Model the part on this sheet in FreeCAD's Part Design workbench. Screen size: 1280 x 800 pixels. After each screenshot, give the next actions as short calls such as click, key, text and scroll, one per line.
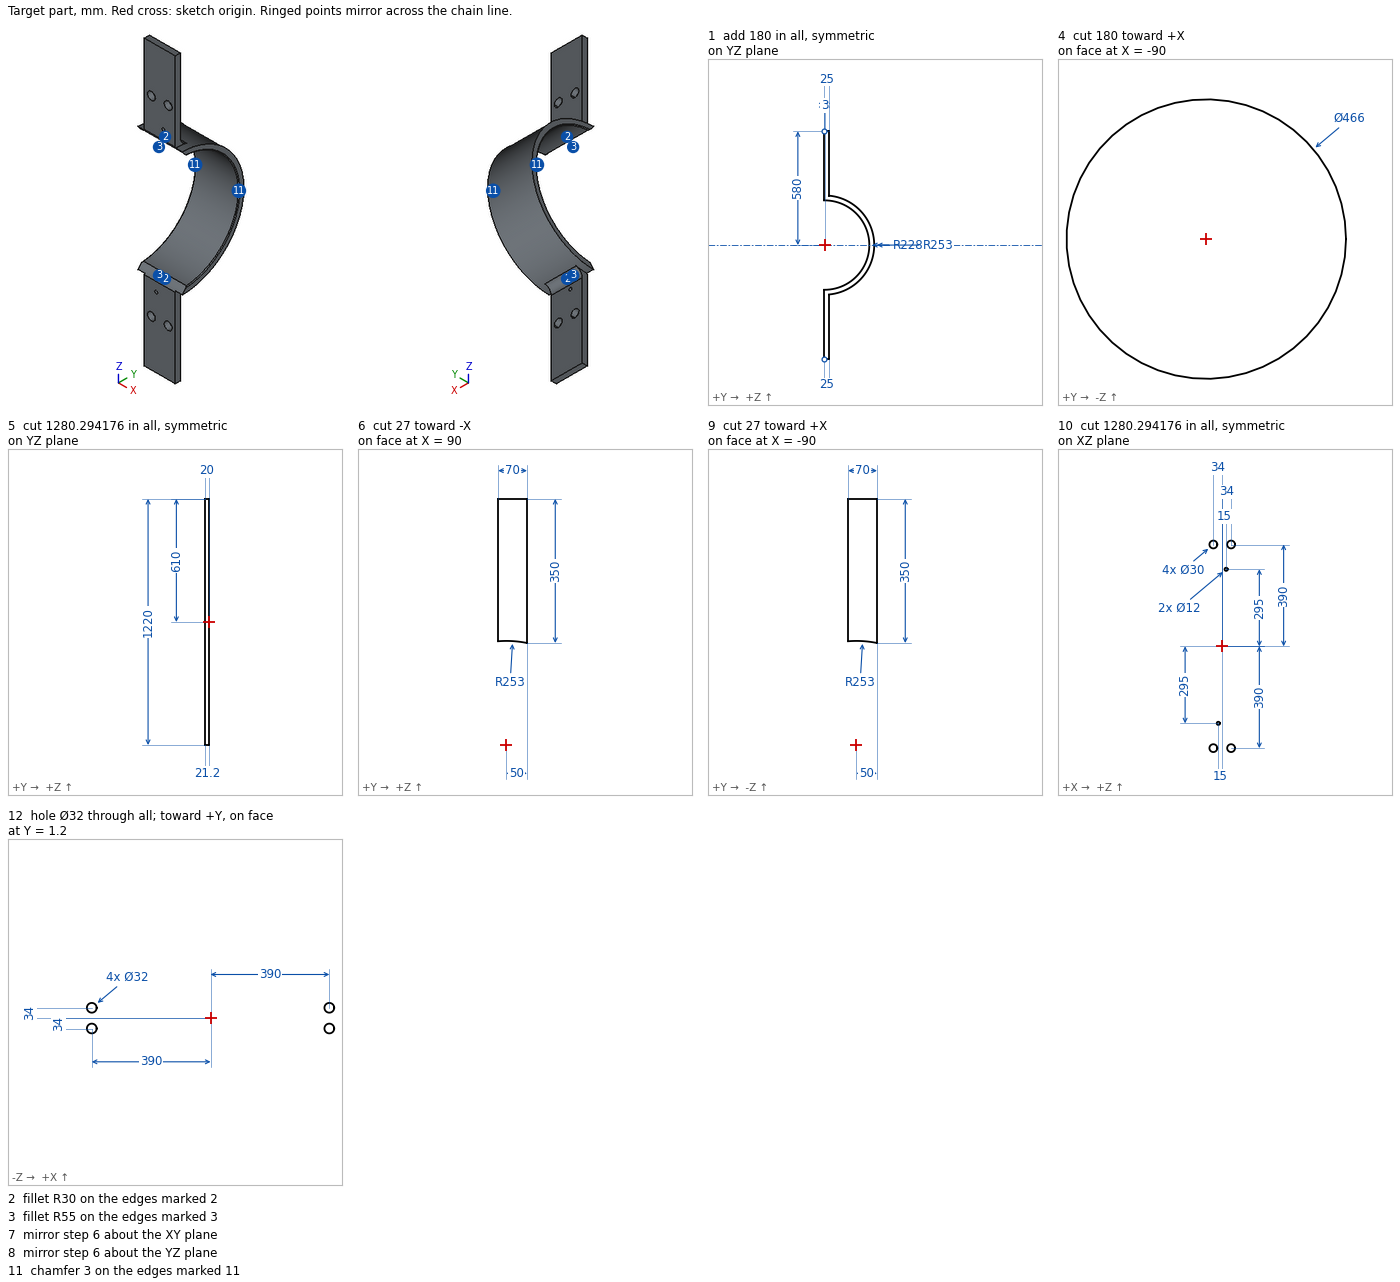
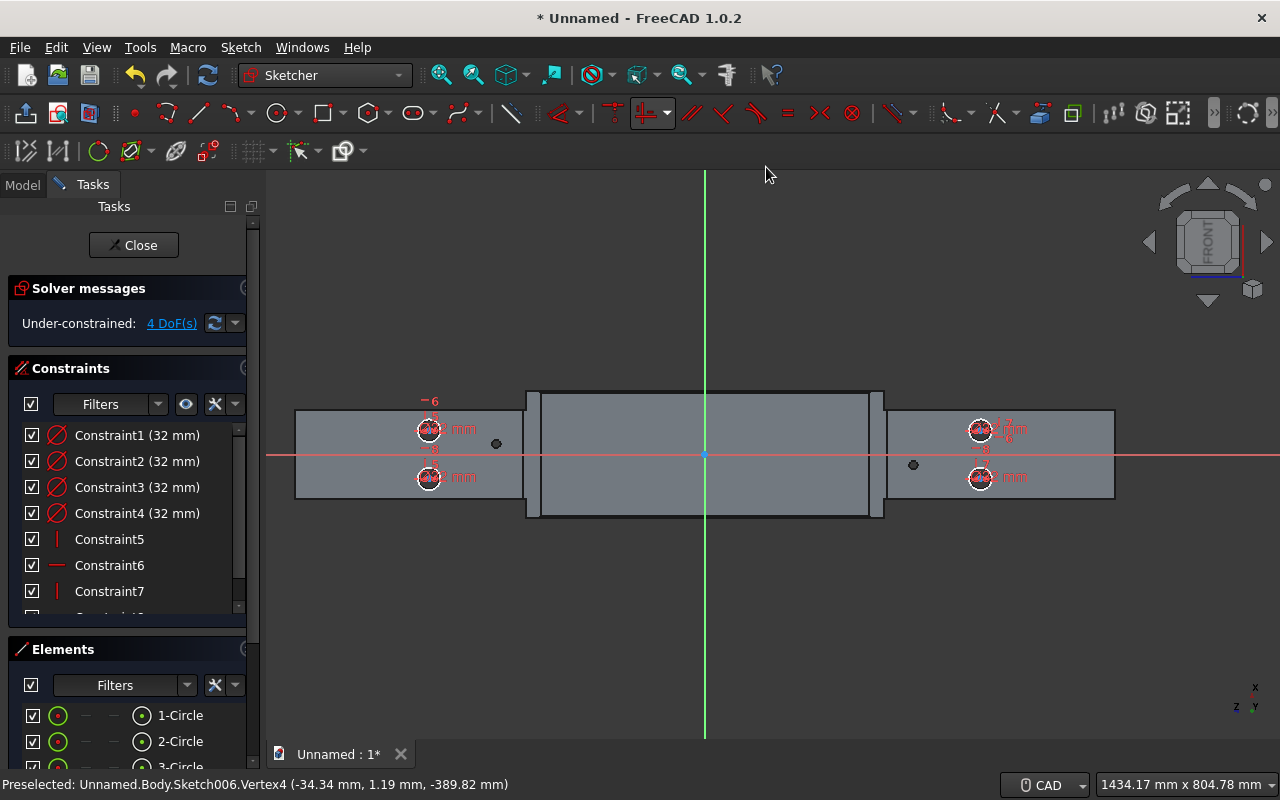
click(558, 114)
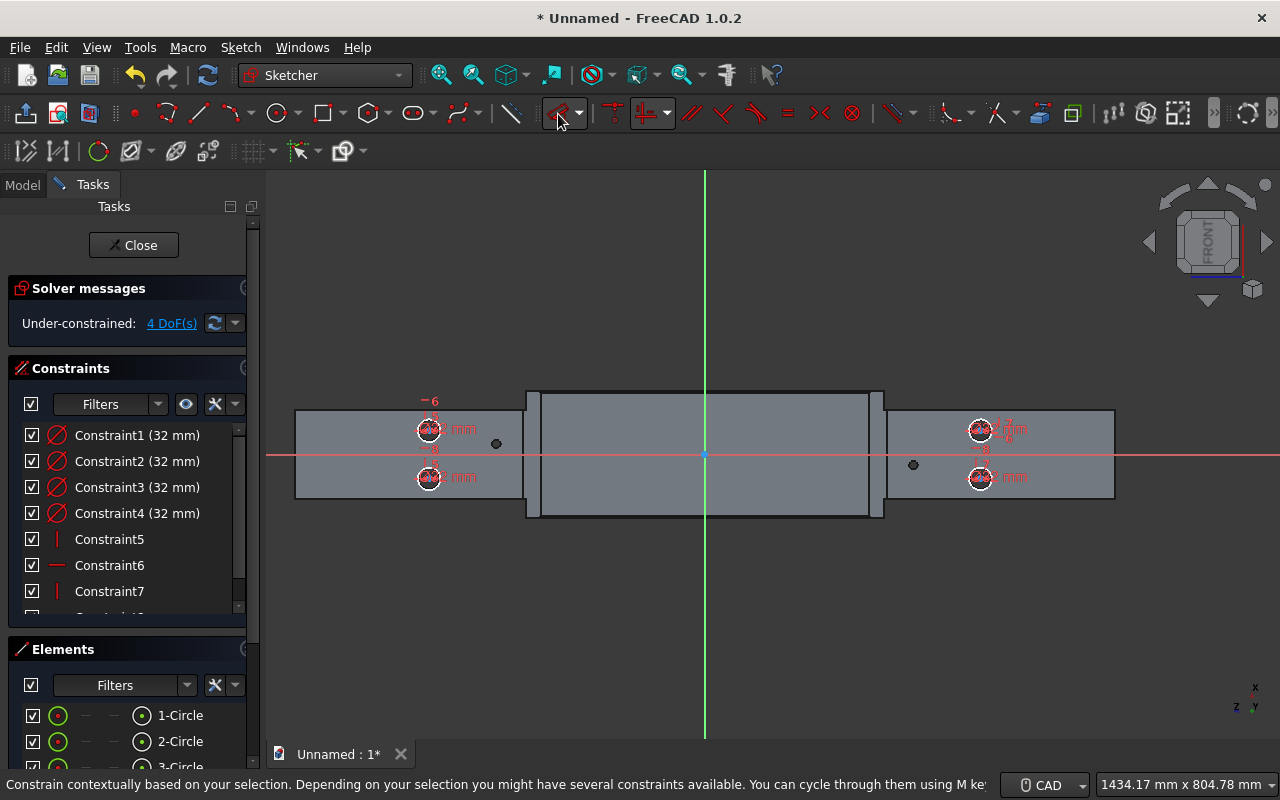
scroll(429, 479, up, 3)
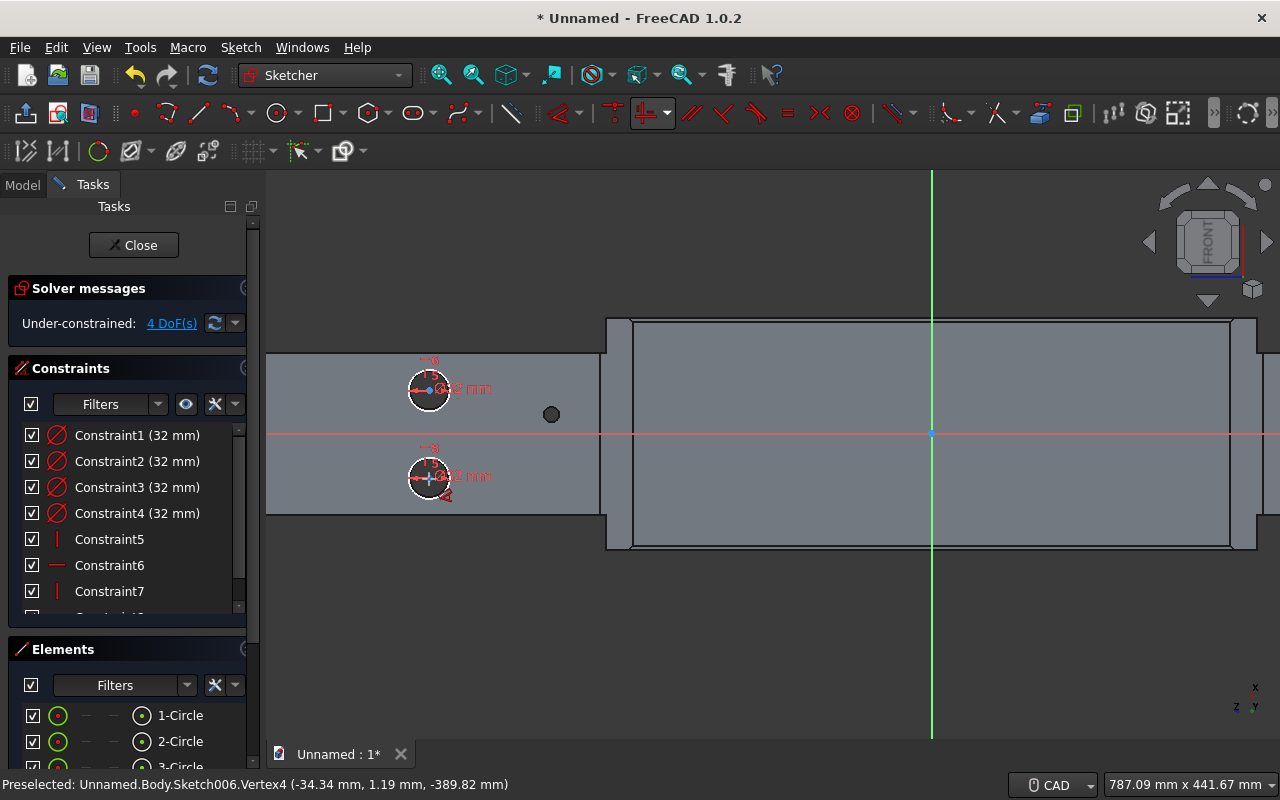
click(429, 478)
click(395, 456)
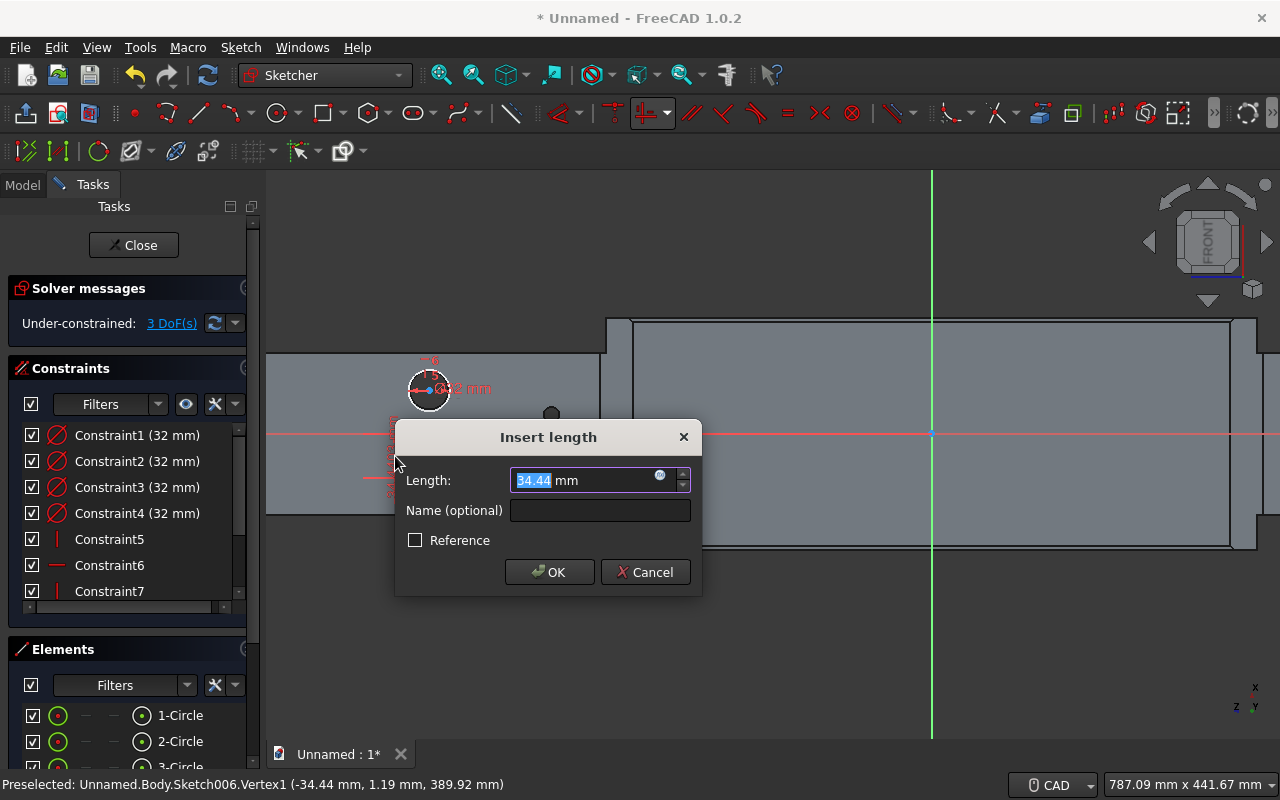
text(34)
key(Return)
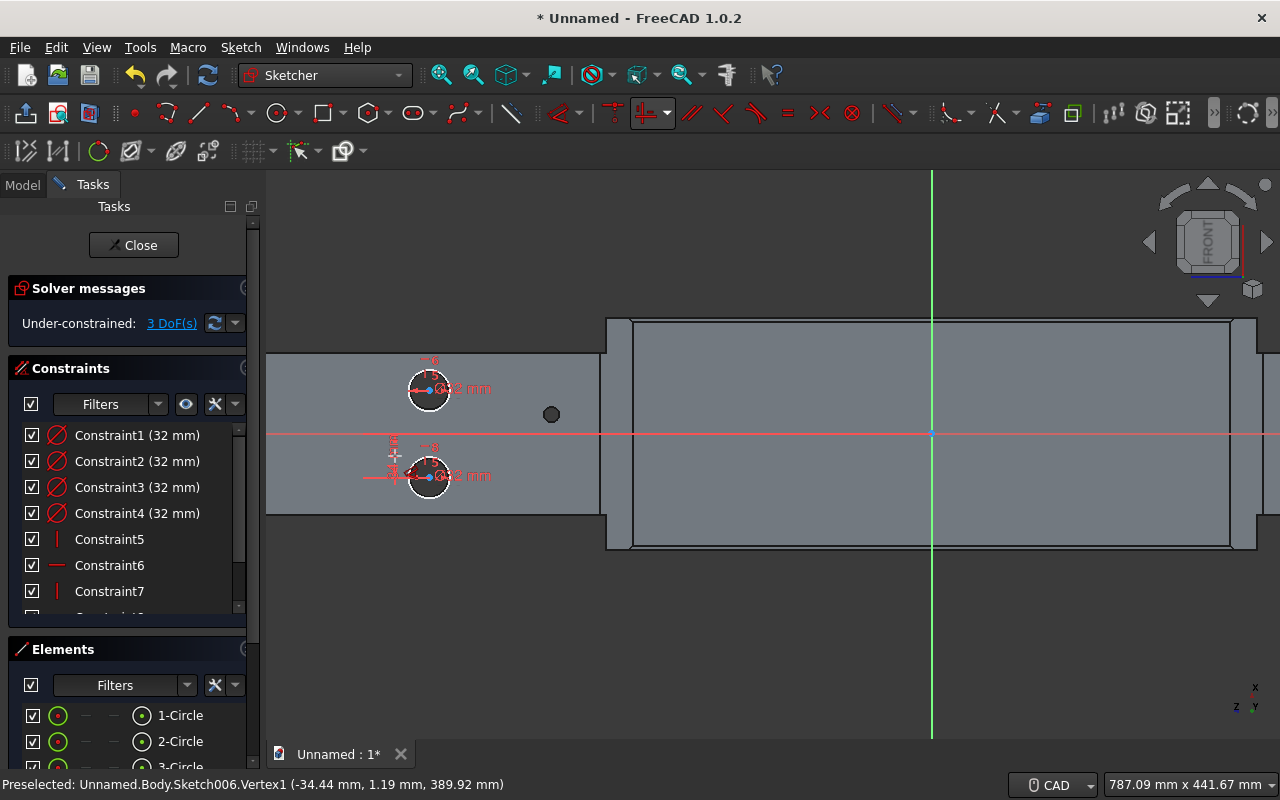
click(429, 391)
click(395, 412)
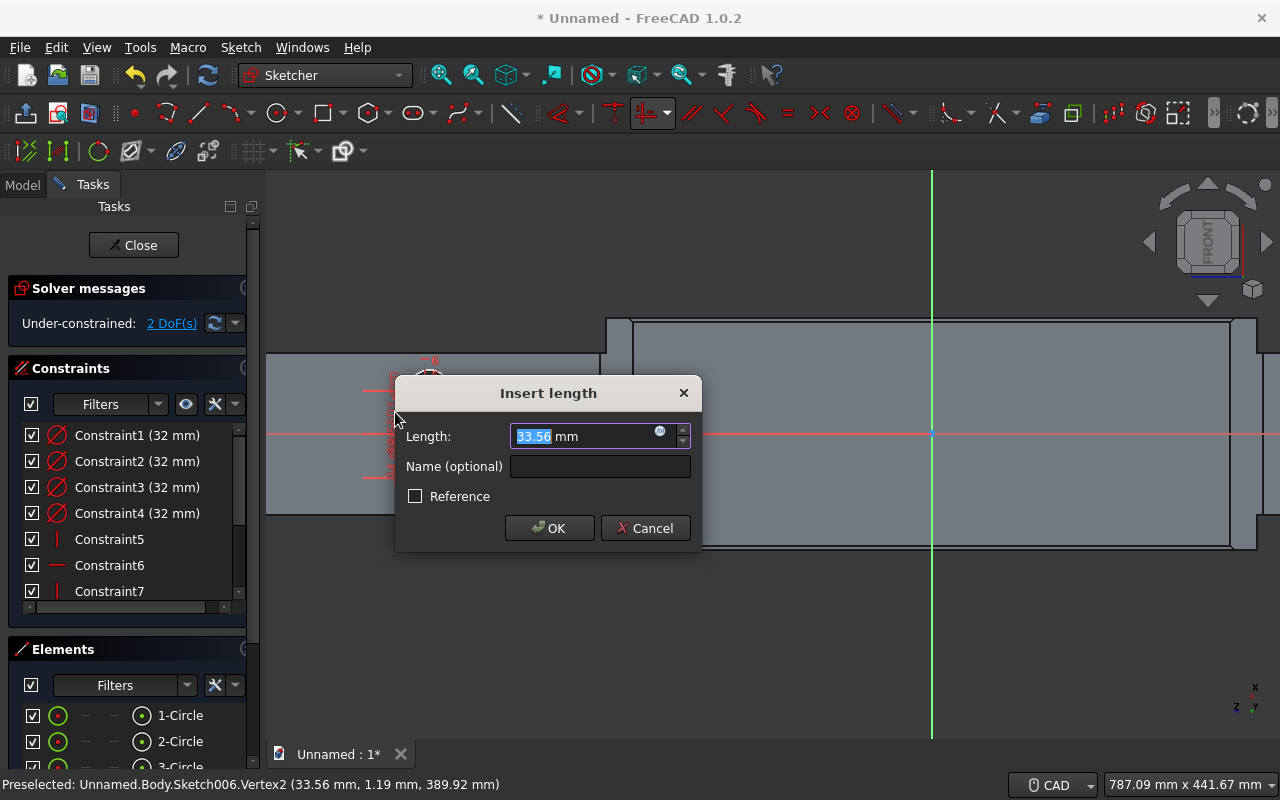
text(34)
key(Return)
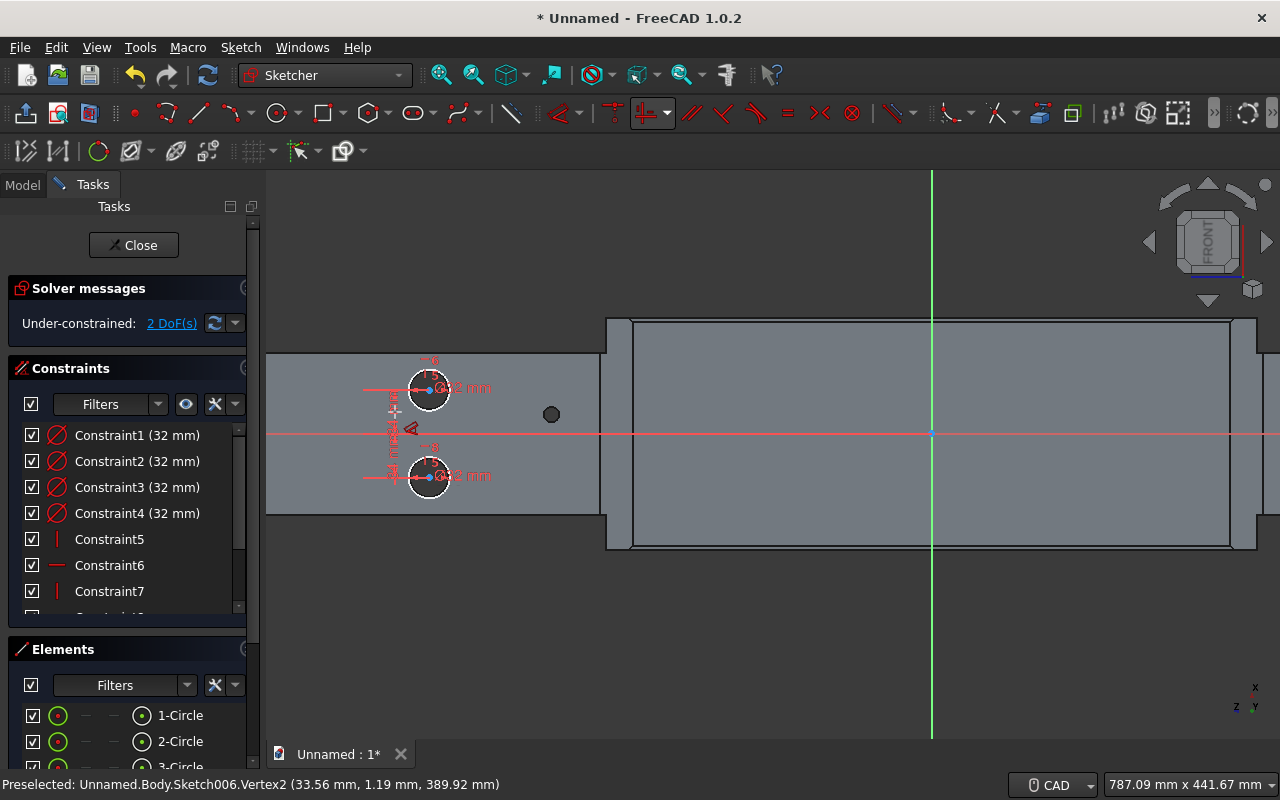
click(429, 478)
click(680, 512)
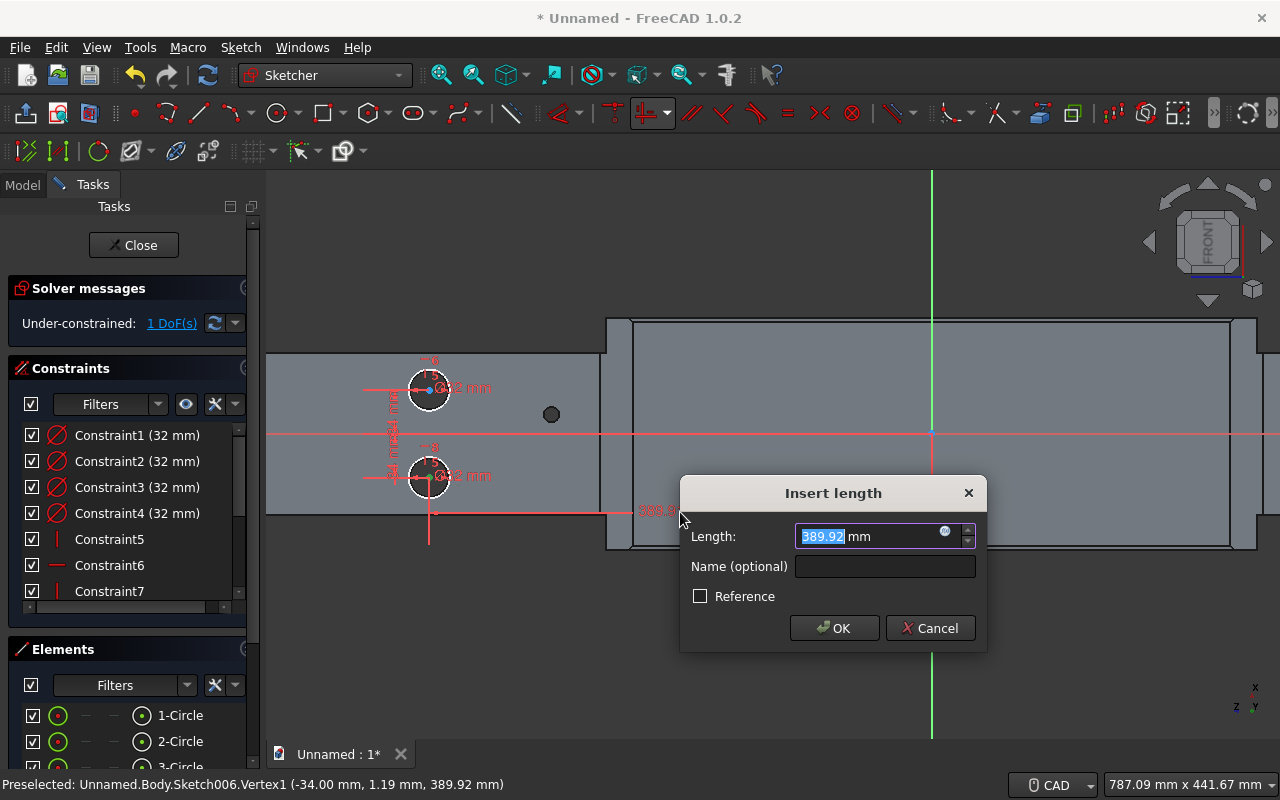
text(390)
key(Return)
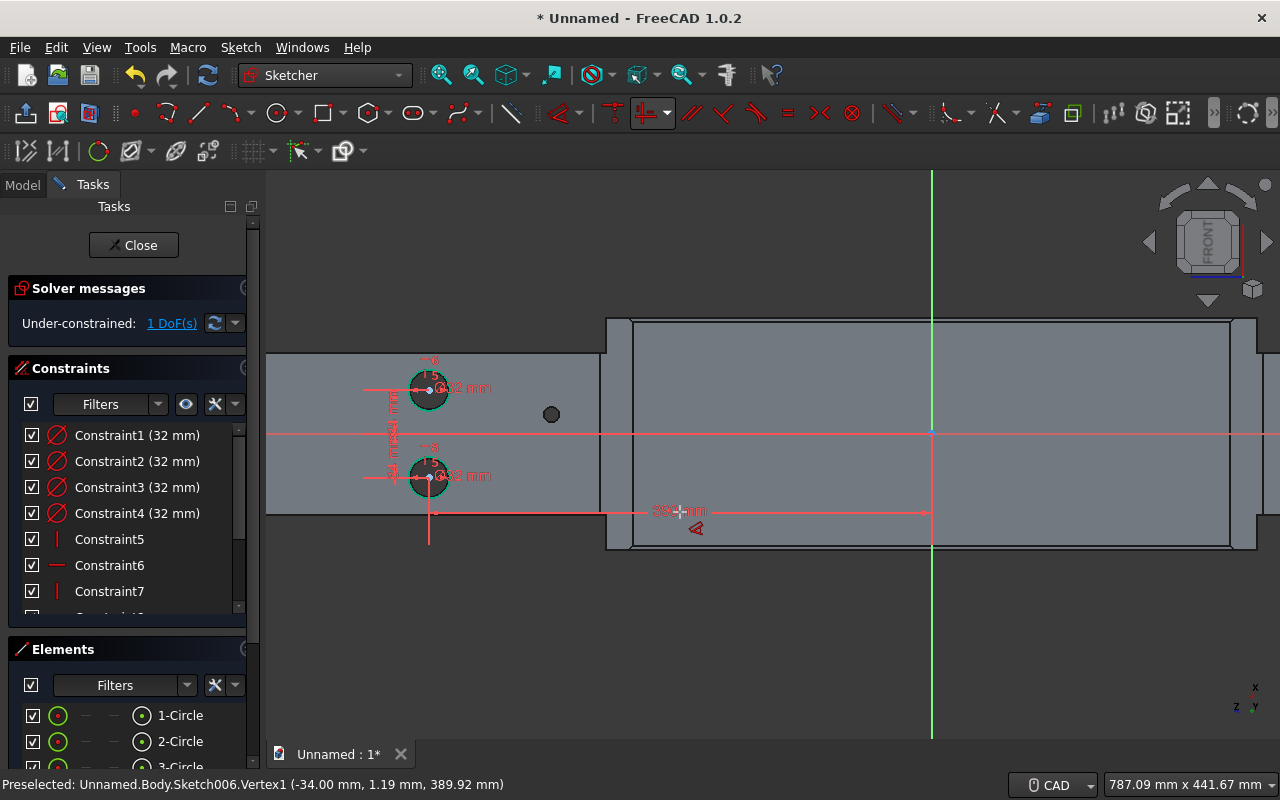
scroll(428, 480, down, 3)